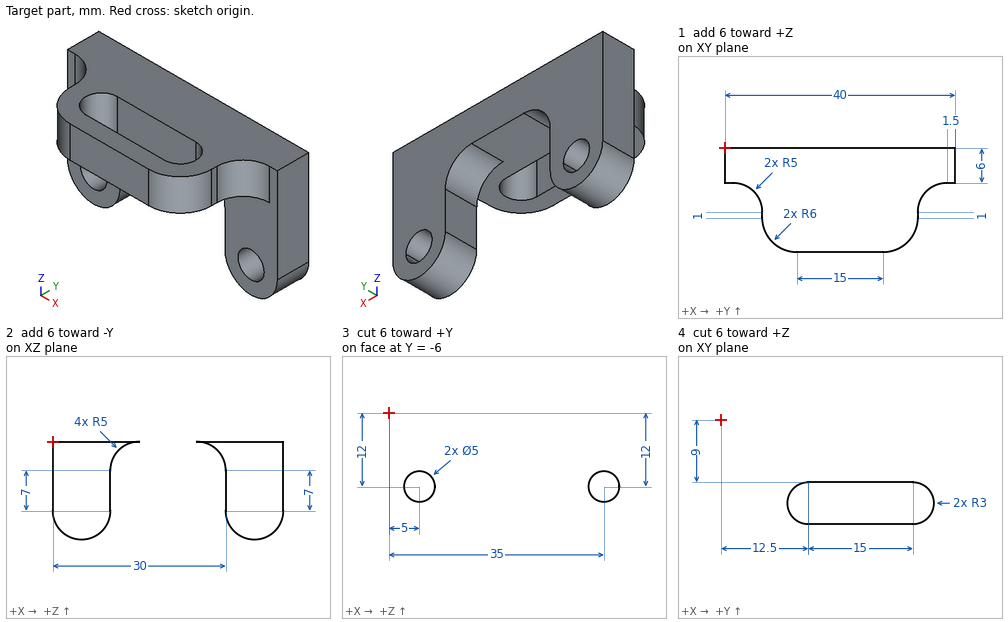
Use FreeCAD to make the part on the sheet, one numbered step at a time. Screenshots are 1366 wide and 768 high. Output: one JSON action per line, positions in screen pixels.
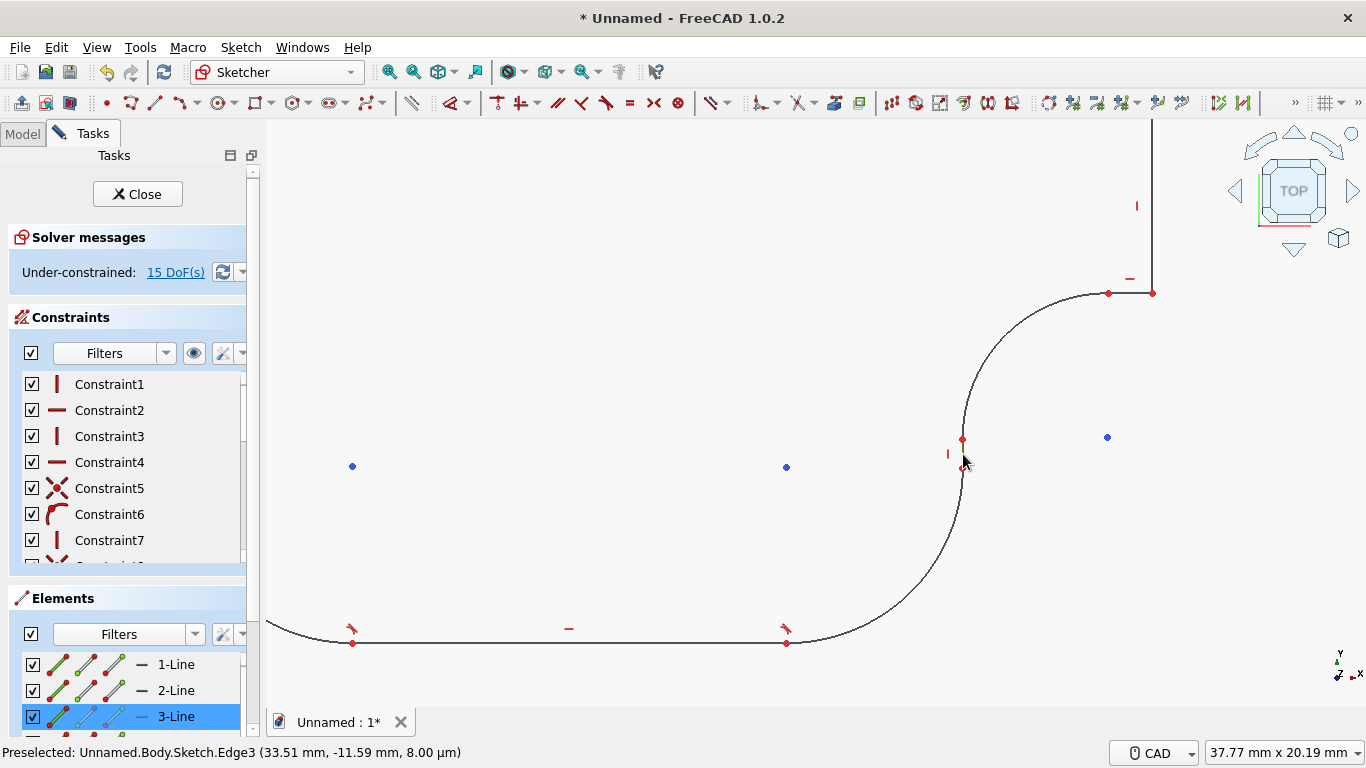
{"action": "left_click", "coordinate": [867, 624]}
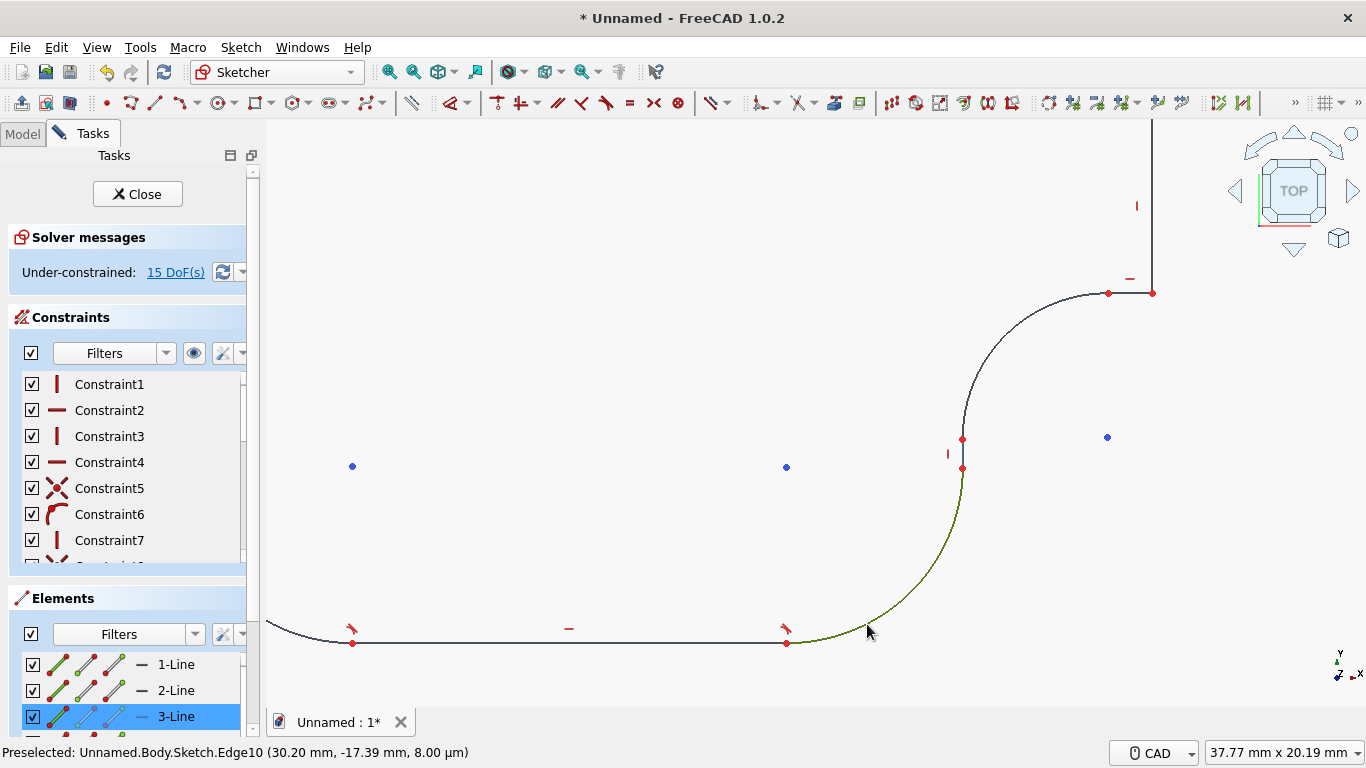
{"action": "key", "text": "t"}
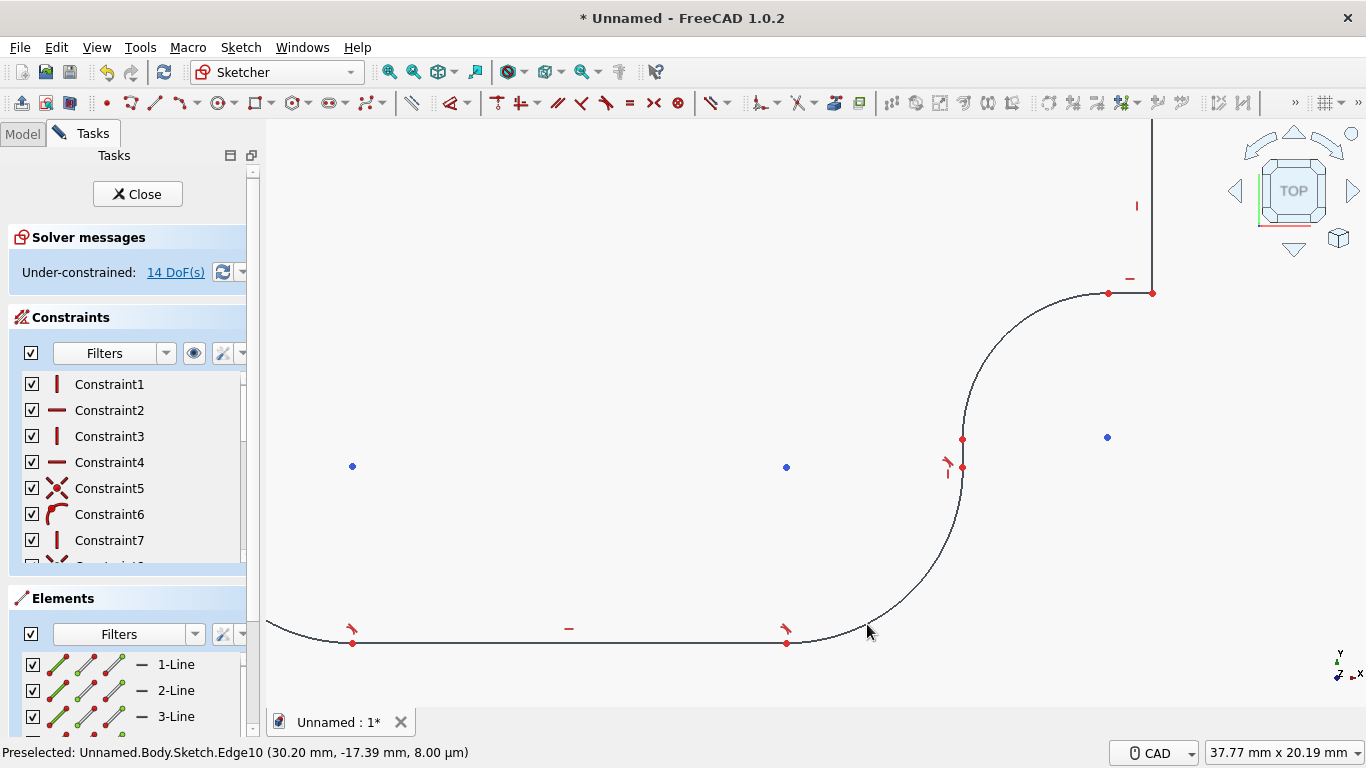
{"action": "scroll", "coordinate": [963, 456], "scroll_direction": "up", "scroll_amount": 2}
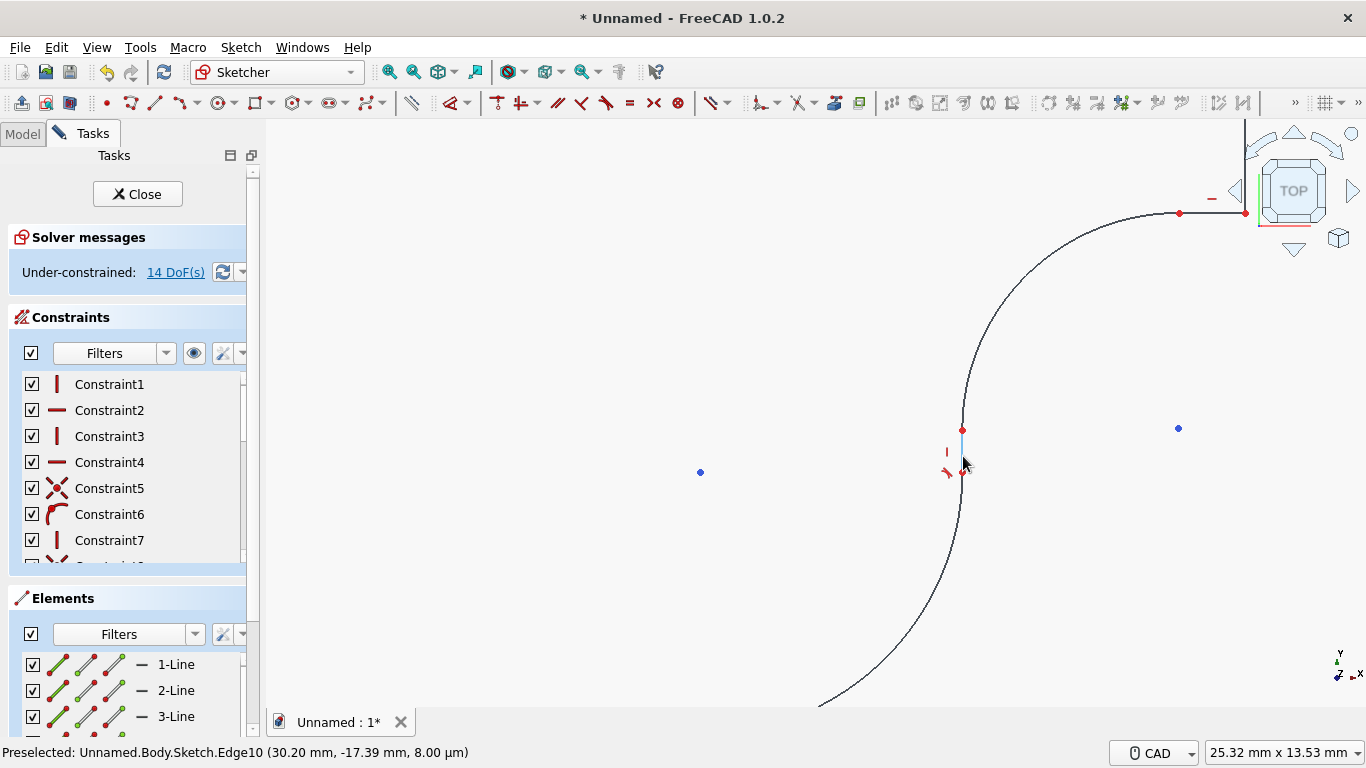
{"action": "left_click", "coordinate": [962, 456]}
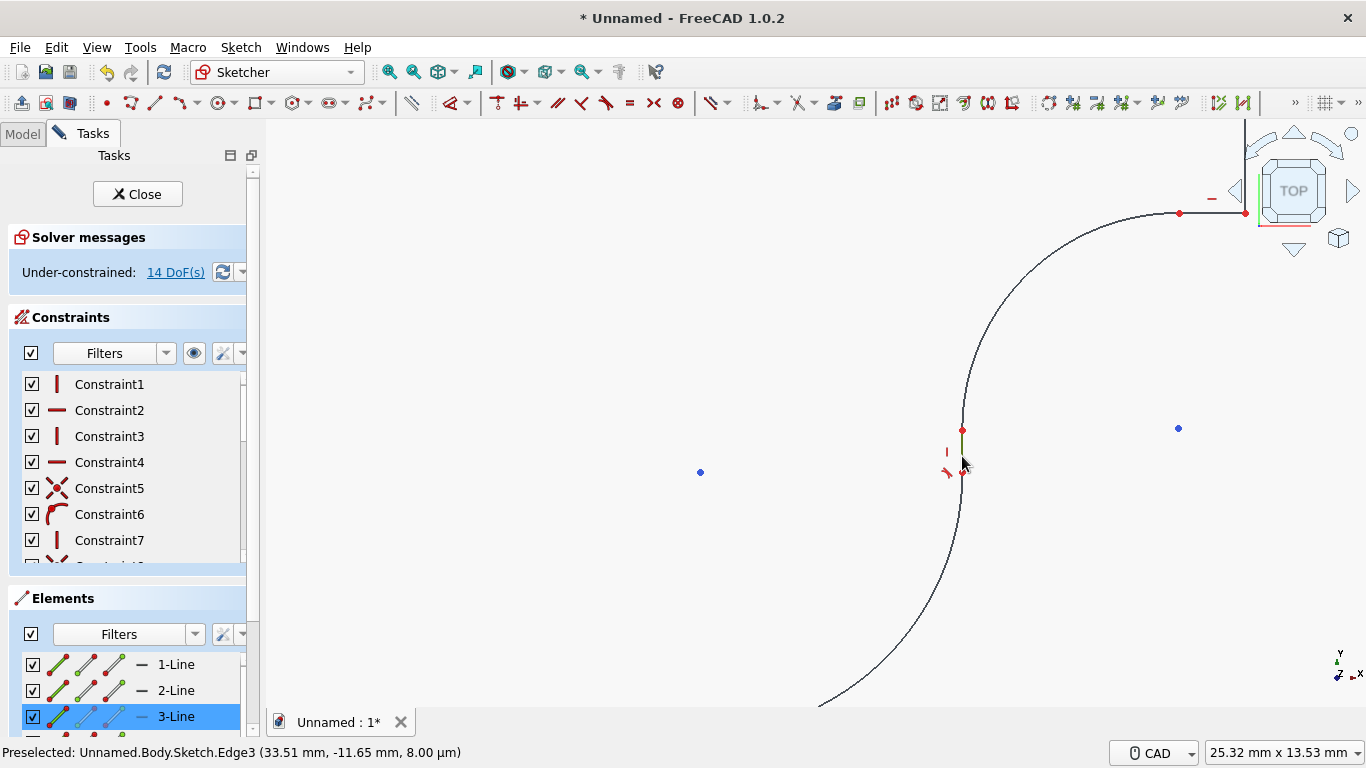
{"action": "left_click", "coordinate": [1081, 236]}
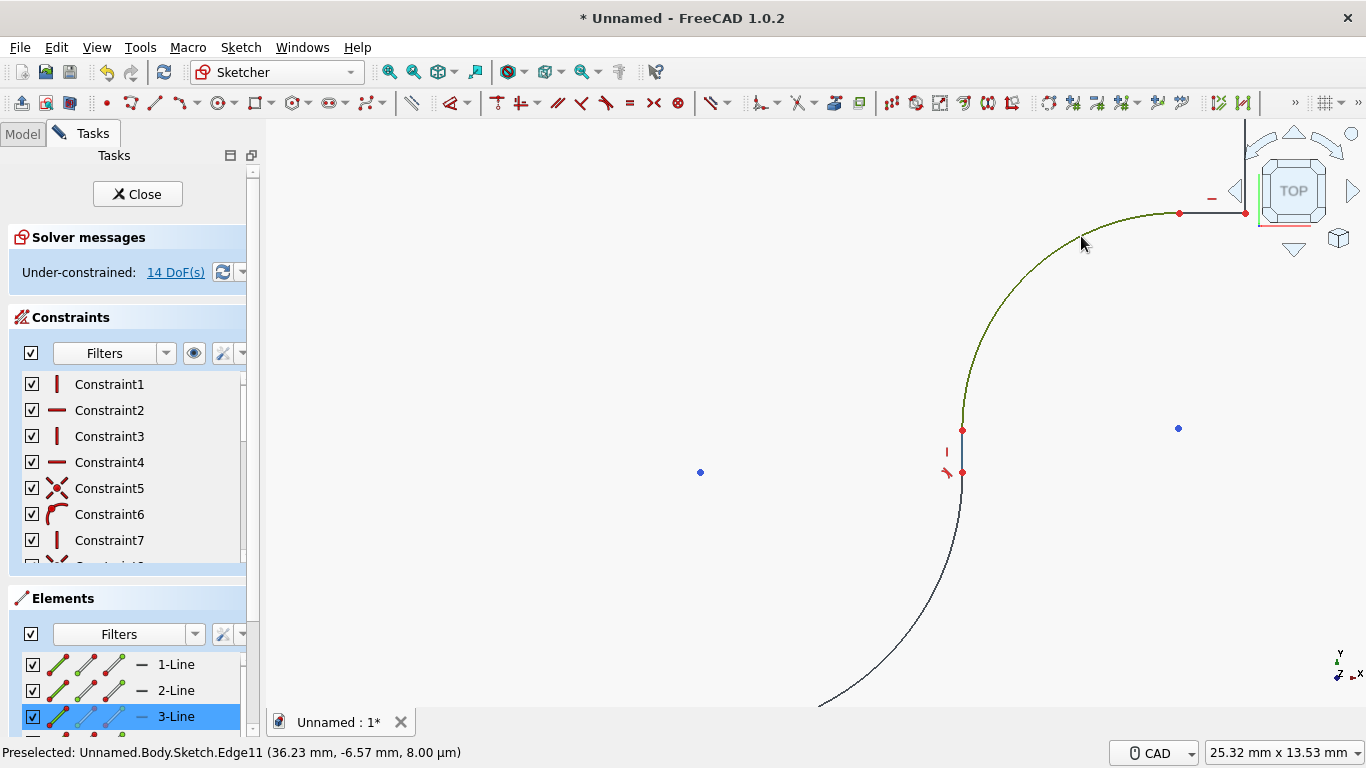
{"action": "left_click", "coordinate": [606, 104]}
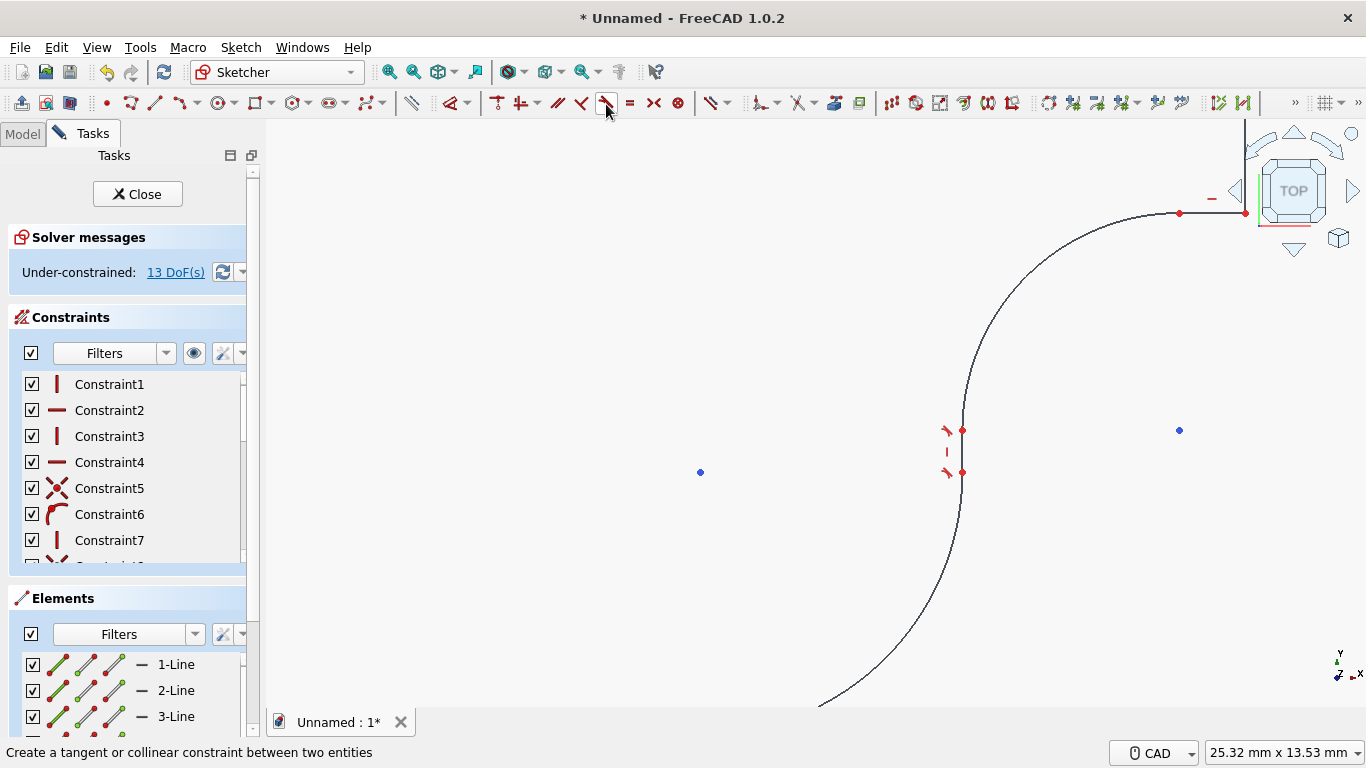
{"action": "left_click", "coordinate": [1199, 213]}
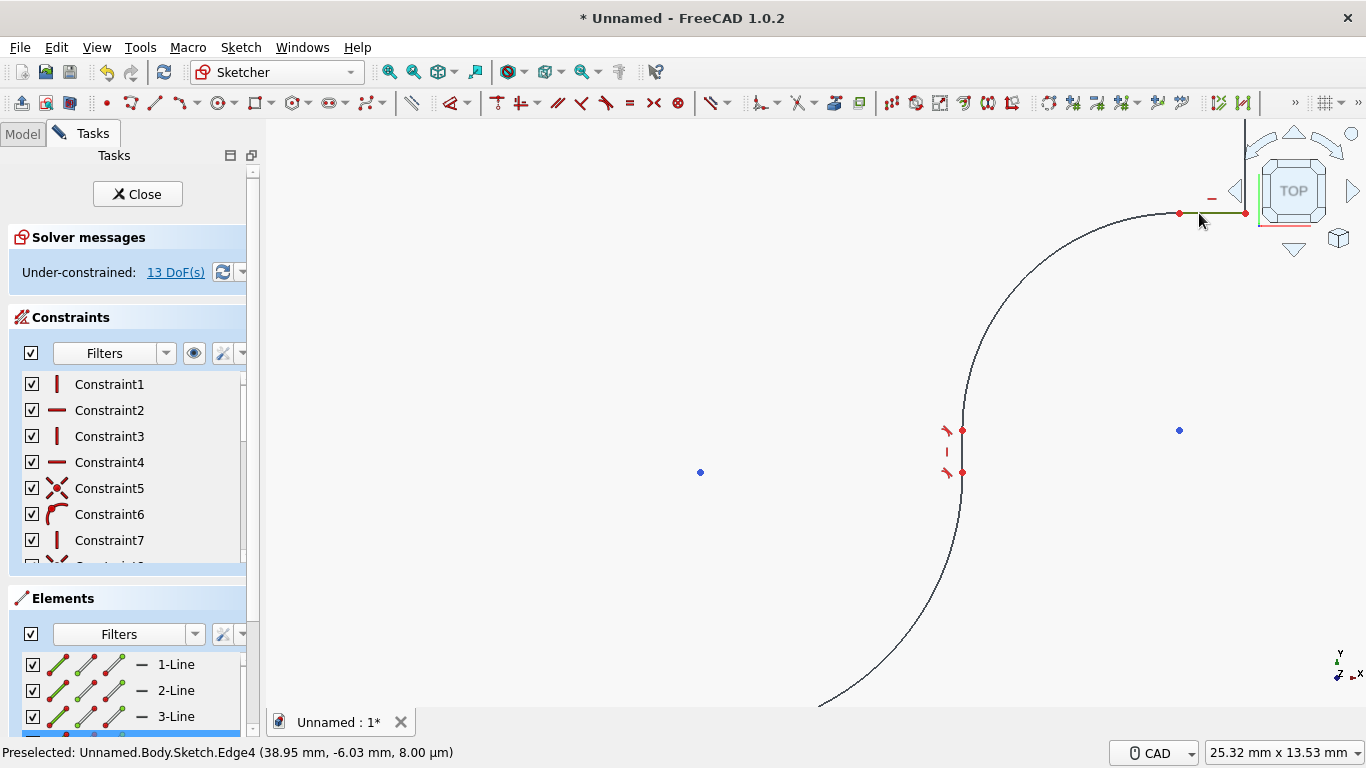
{"action": "left_click", "coordinate": [1081, 237]}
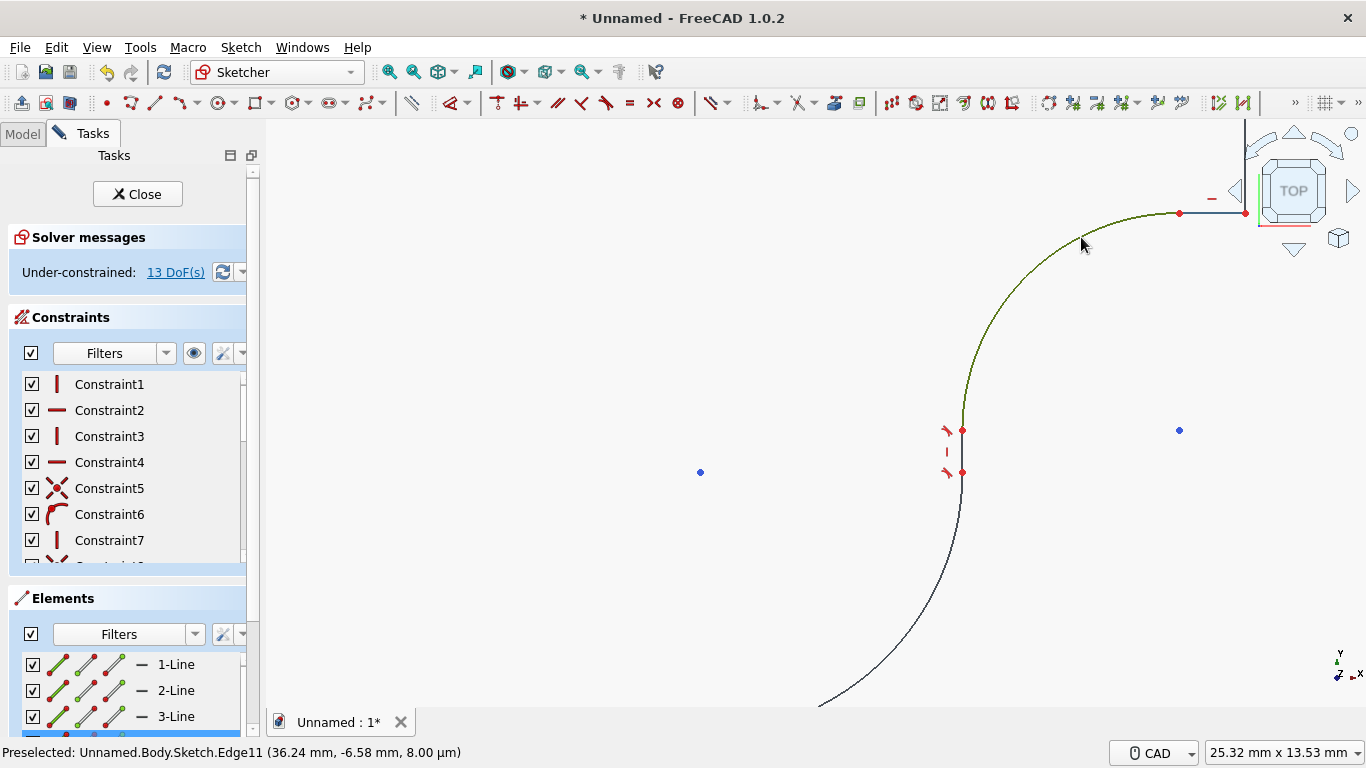
{"action": "key", "text": "t"}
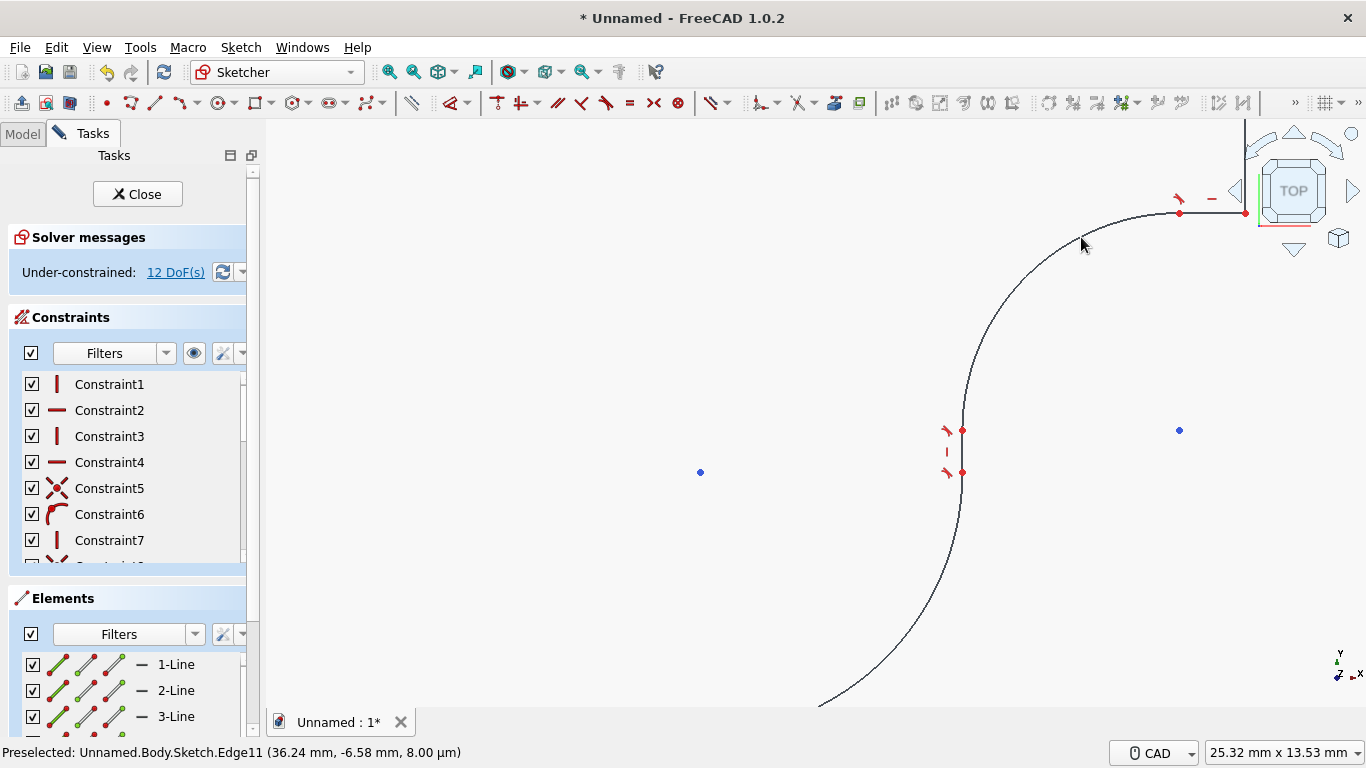
{"action": "scroll", "coordinate": [964, 454], "scroll_direction": "down", "scroll_amount": 5}